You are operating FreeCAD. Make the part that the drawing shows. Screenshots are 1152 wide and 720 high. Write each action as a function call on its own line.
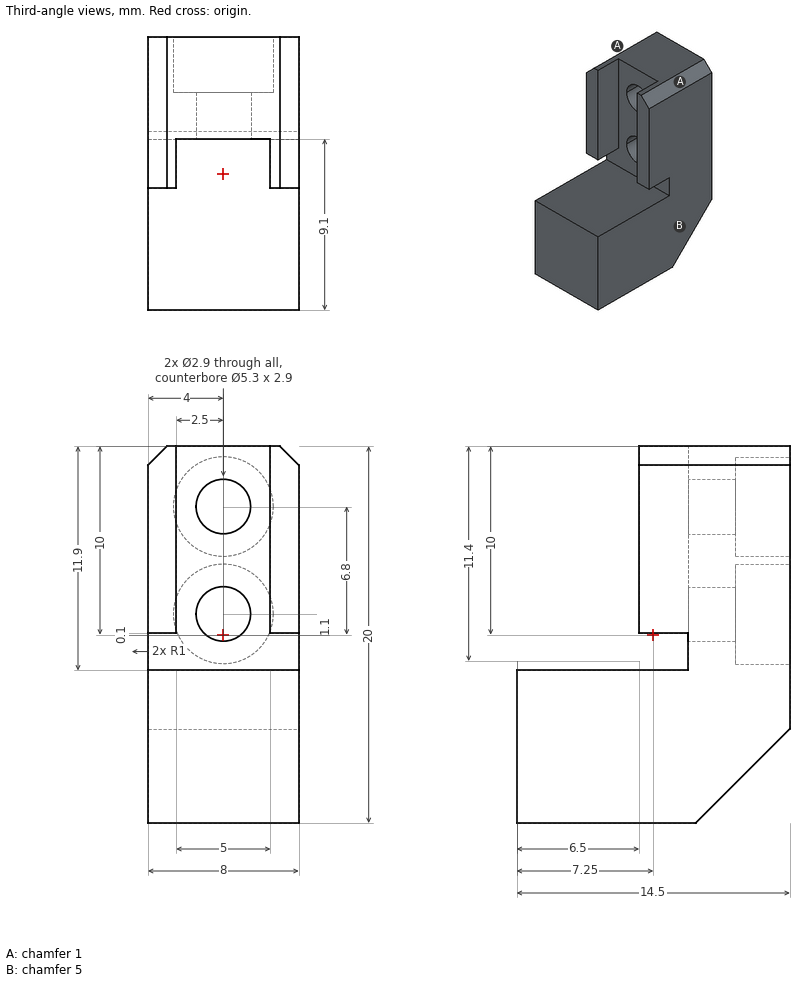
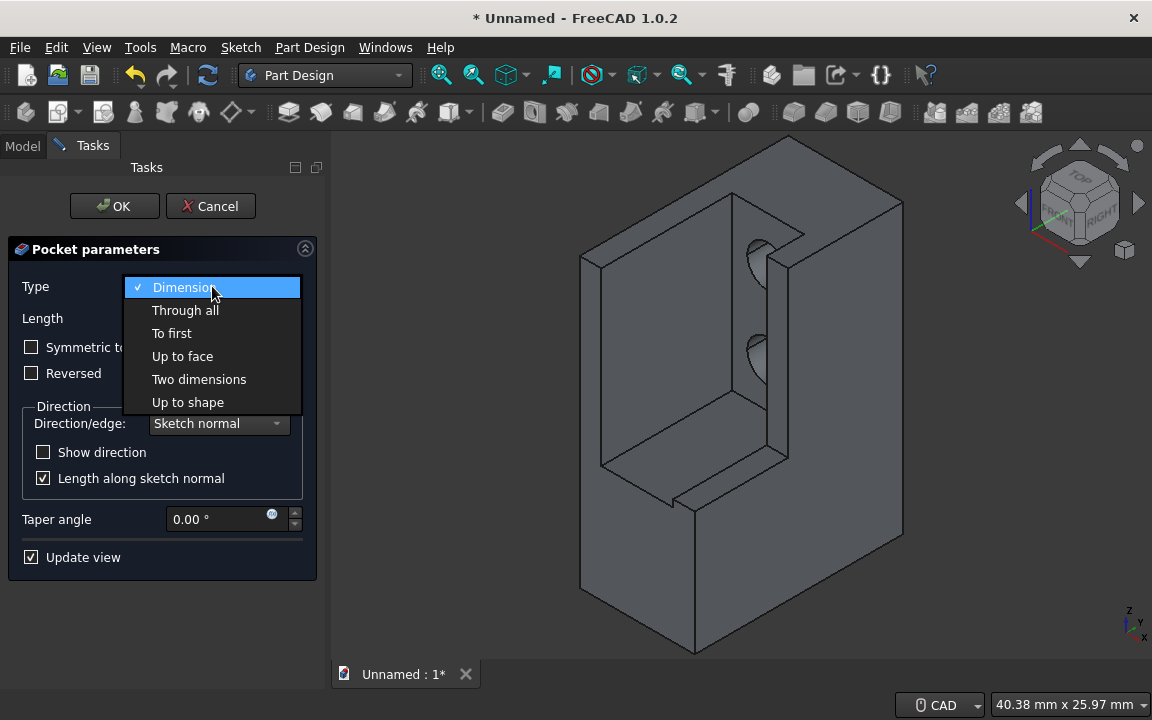
click(212, 310)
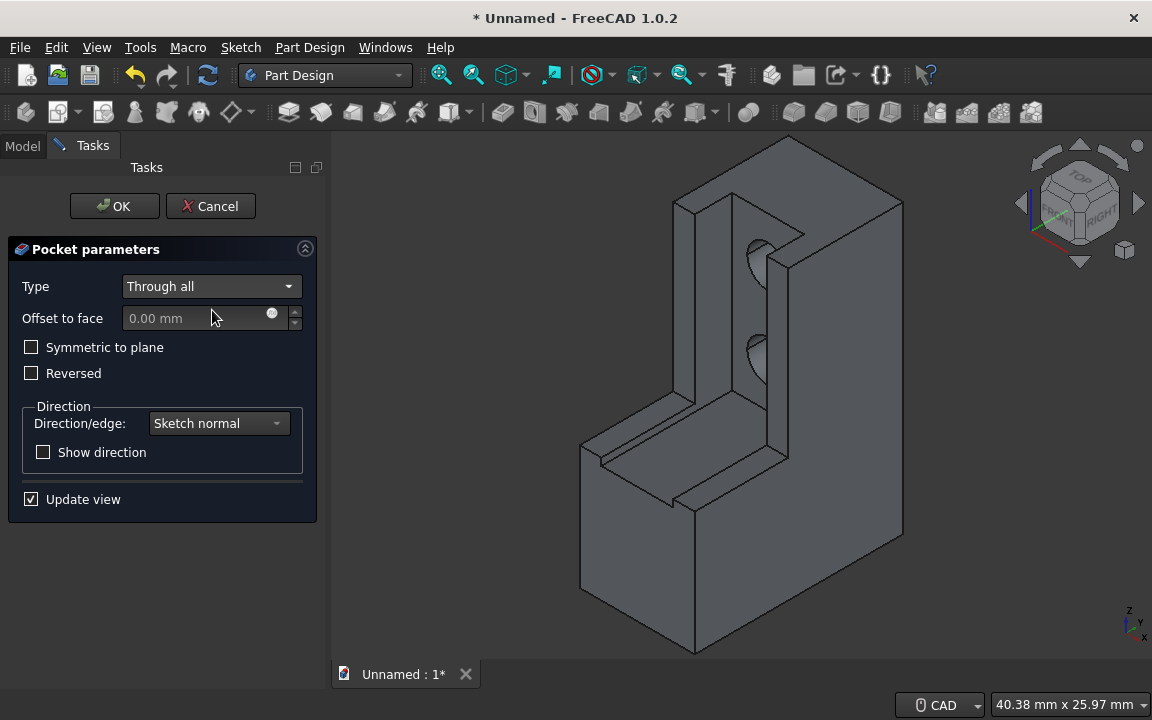
click(115, 206)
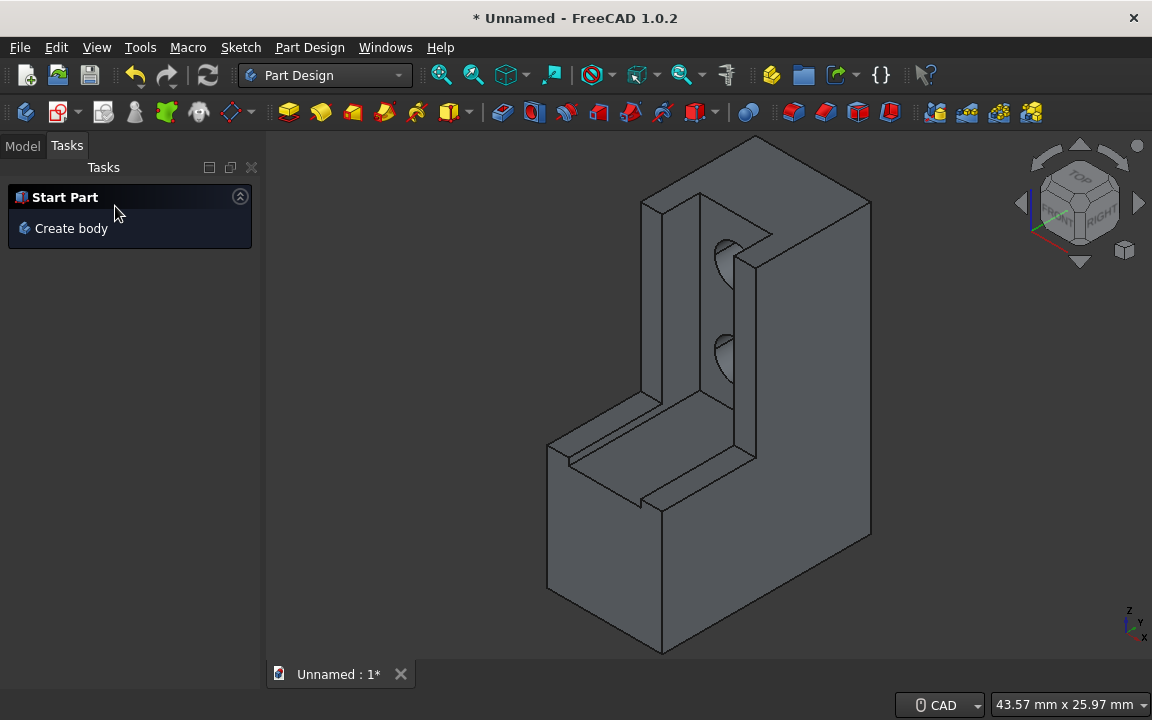
click(813, 234)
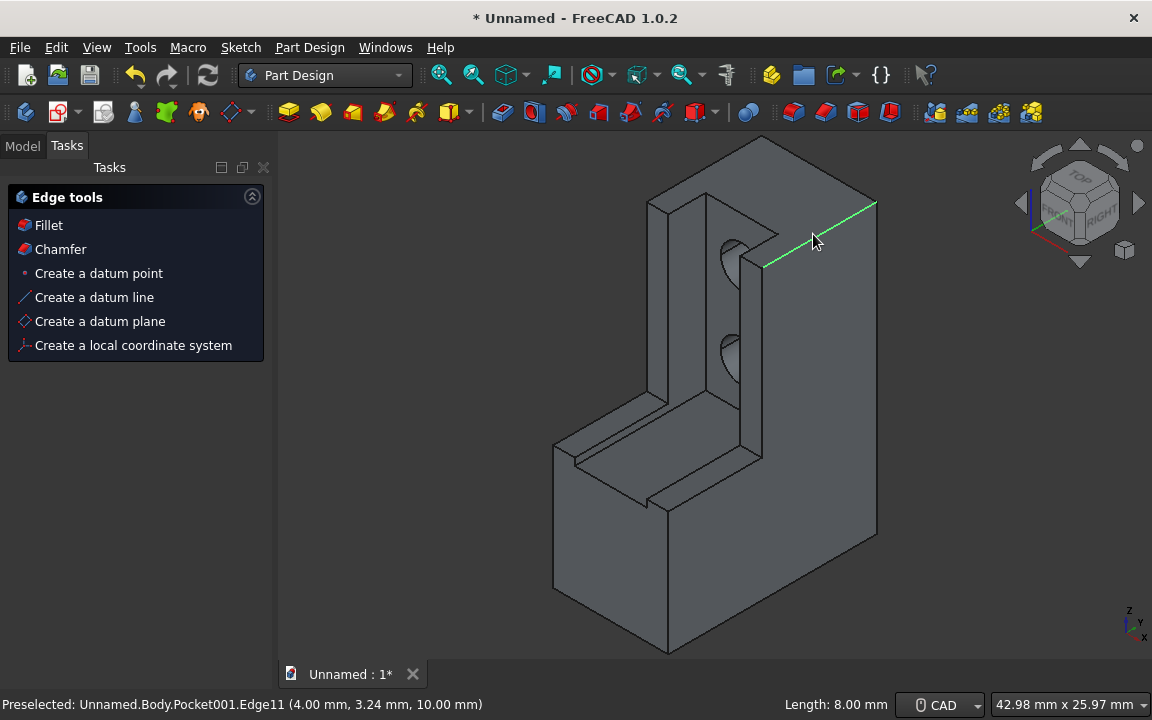
key(2)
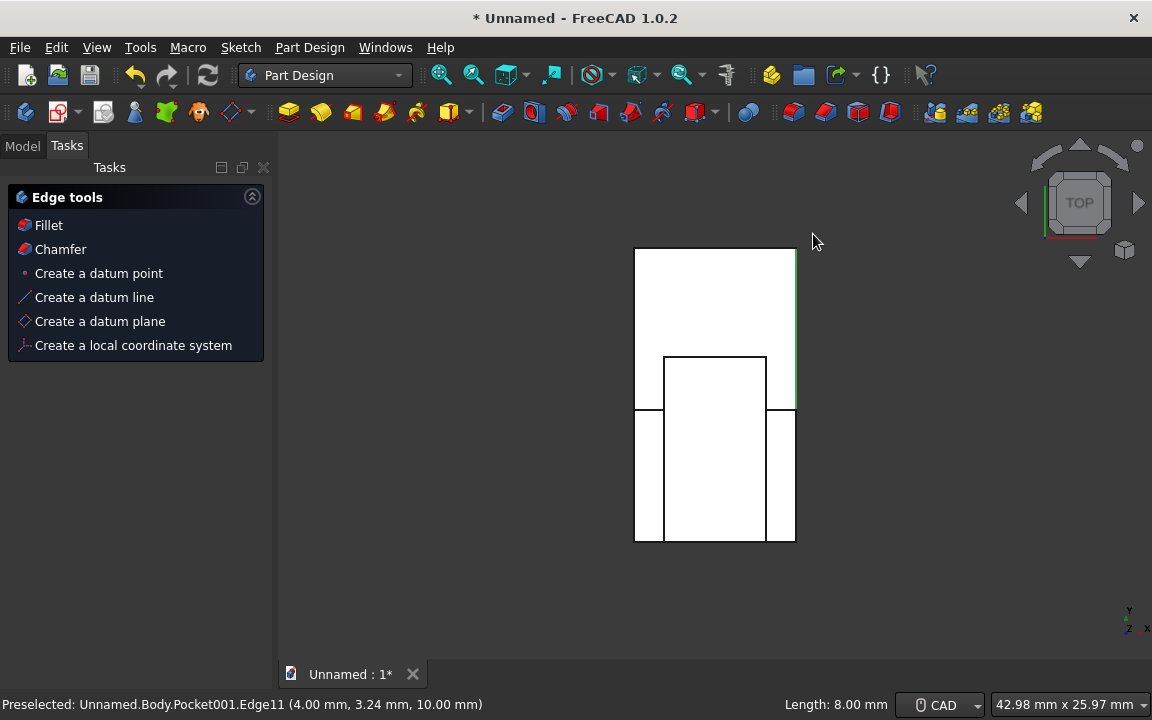
click(634, 328, ctrl)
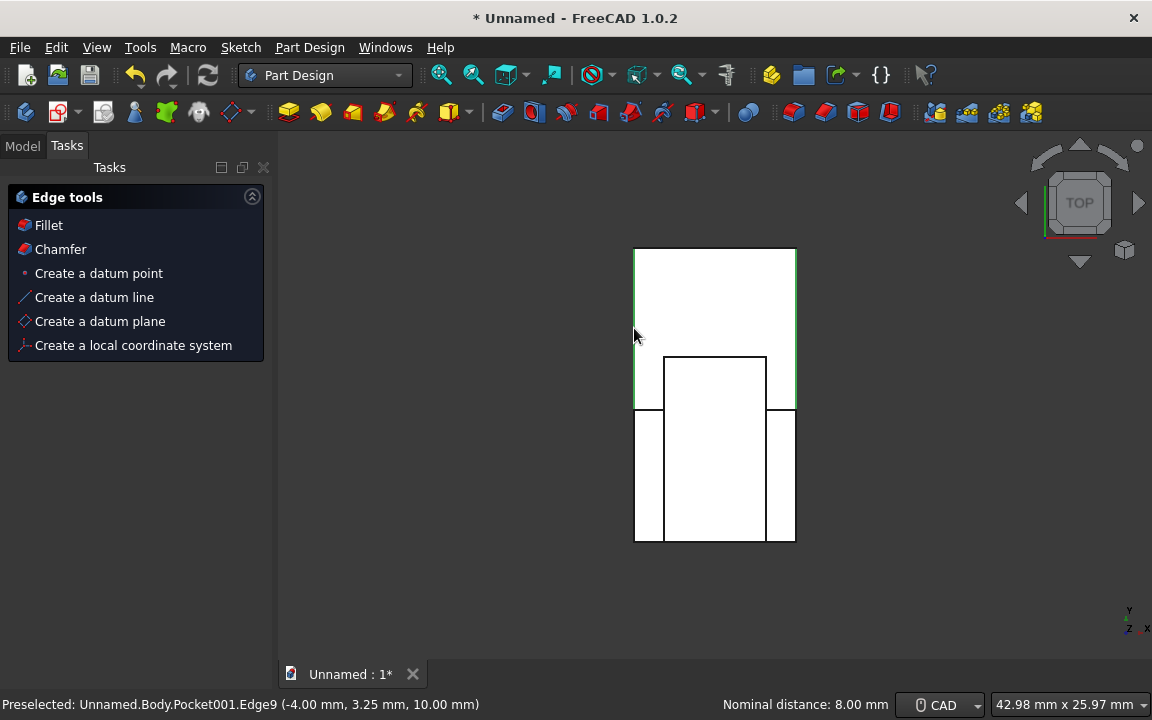
click(826, 112)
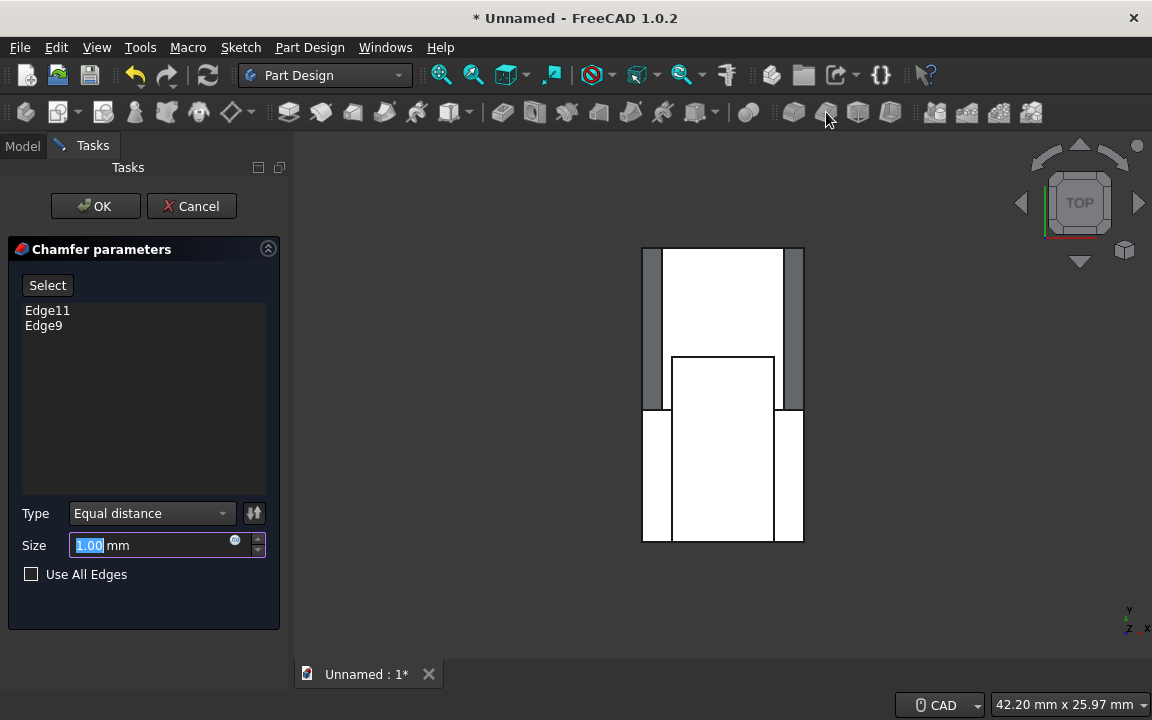
text(1)
key(Tab)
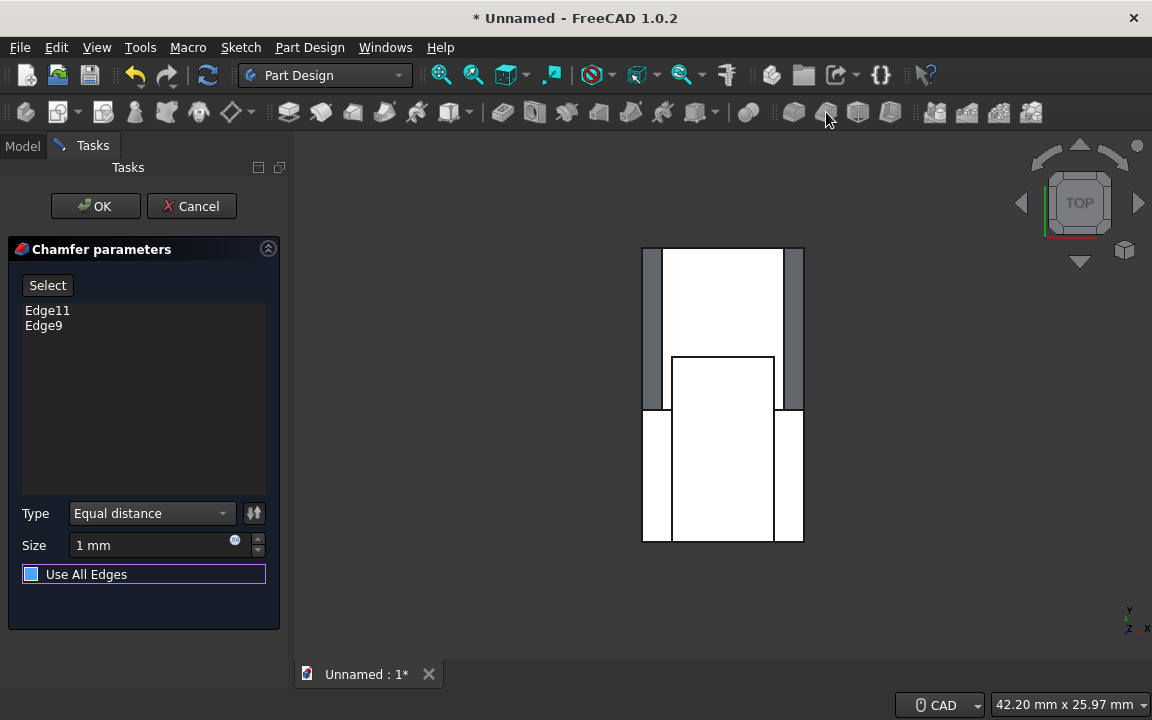
click(96, 206)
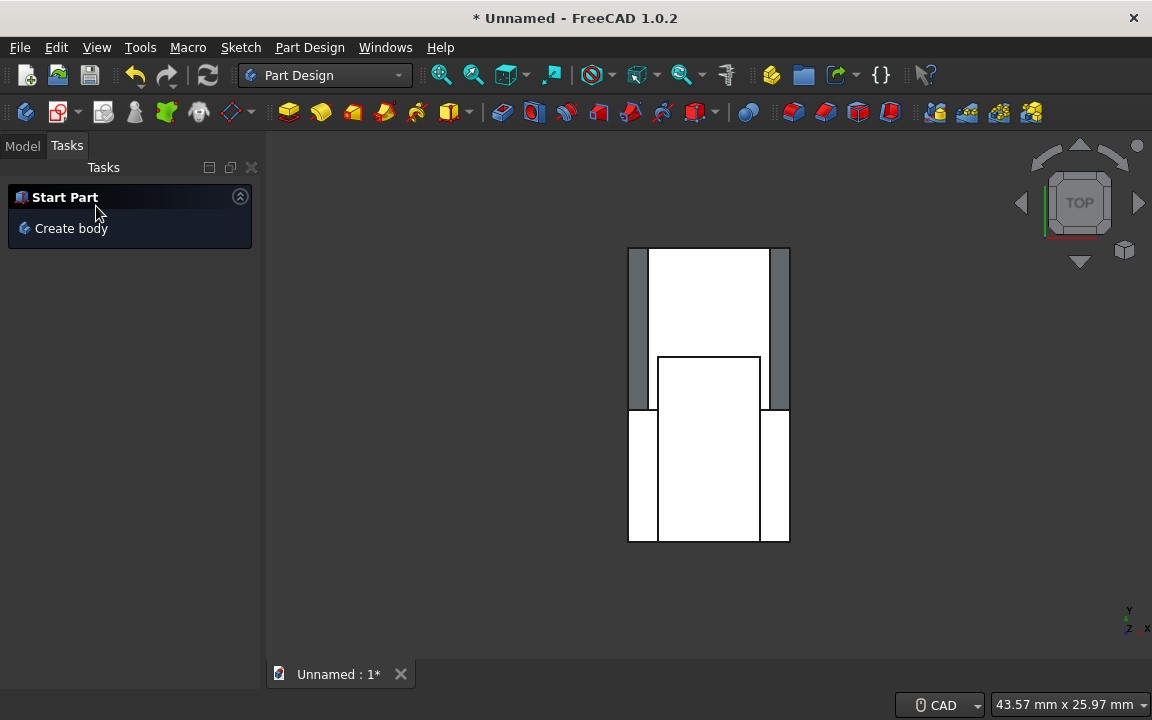
key(0)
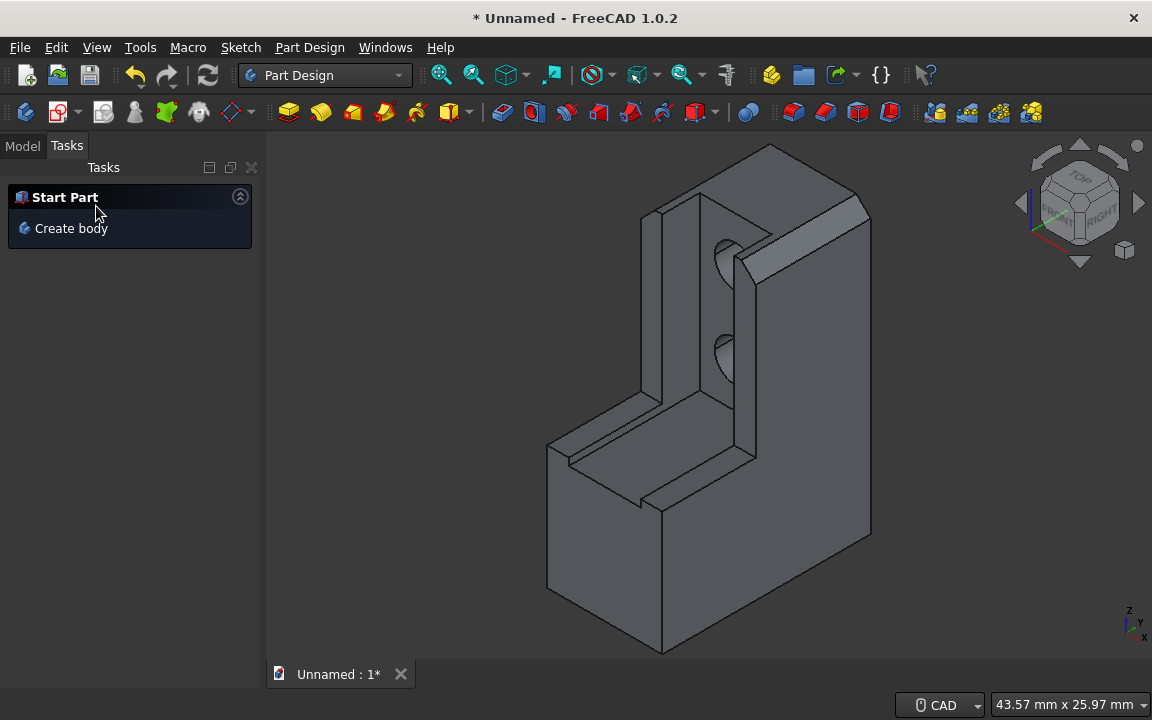
key(2)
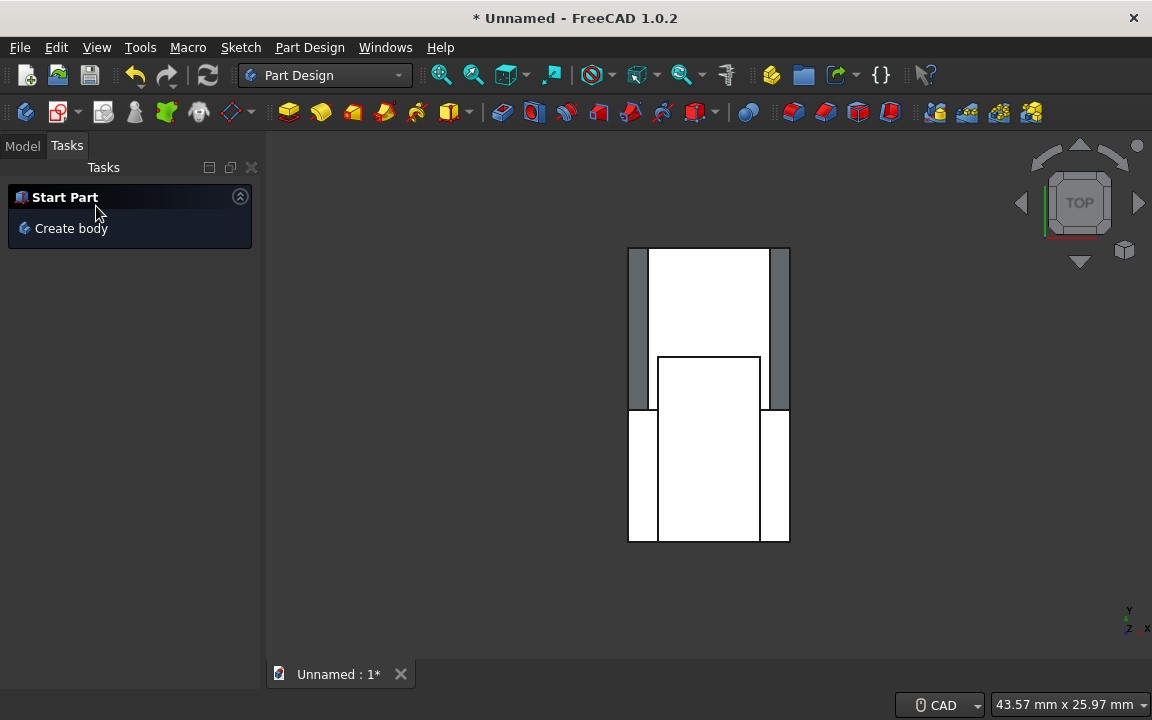
key(1)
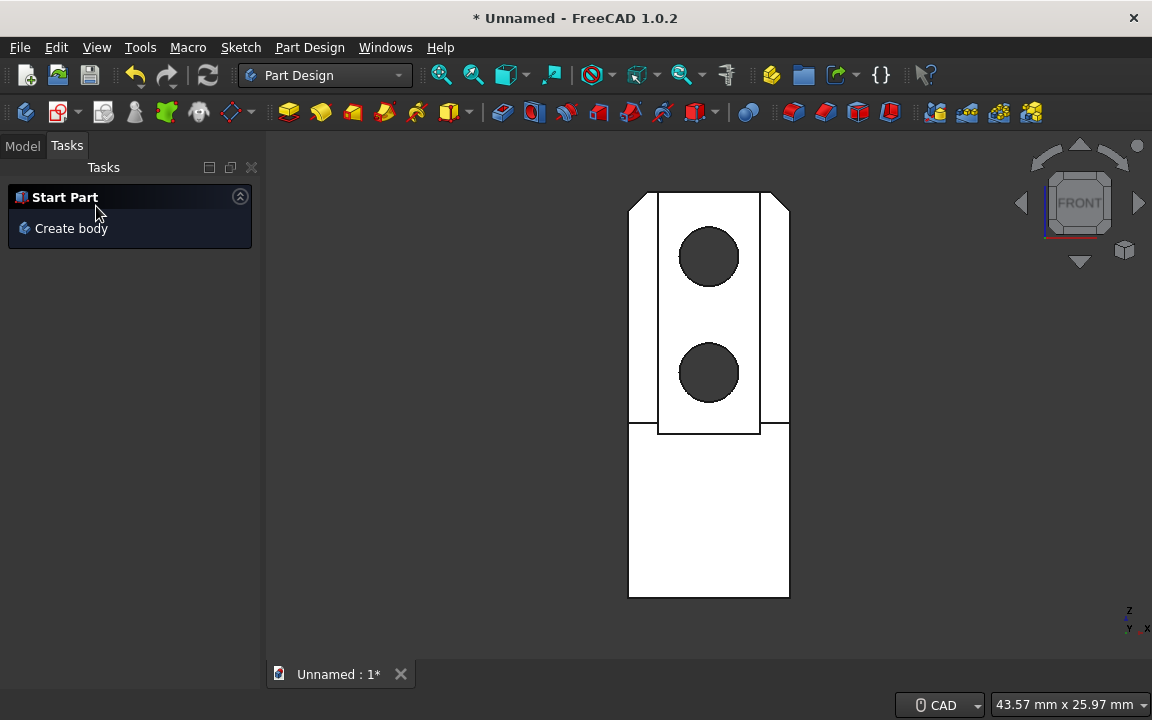
key(3)